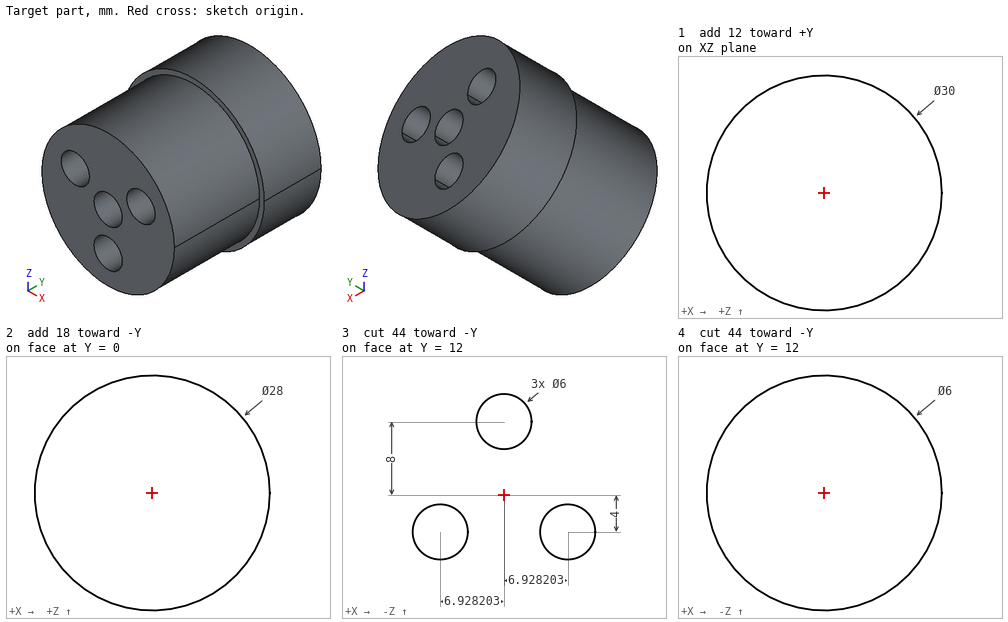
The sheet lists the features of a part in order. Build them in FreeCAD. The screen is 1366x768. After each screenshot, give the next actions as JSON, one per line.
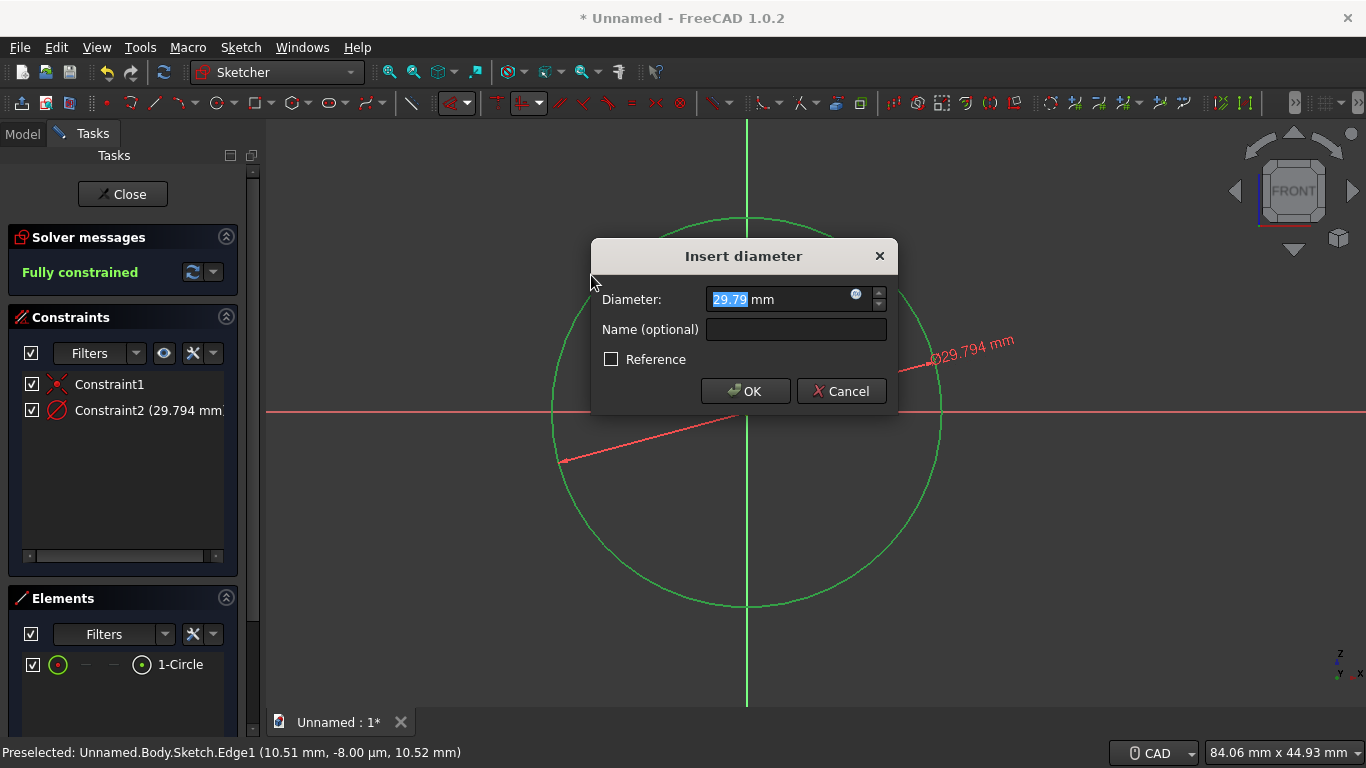
{"action": "type", "text": "30"}
{"action": "key", "text": "Return"}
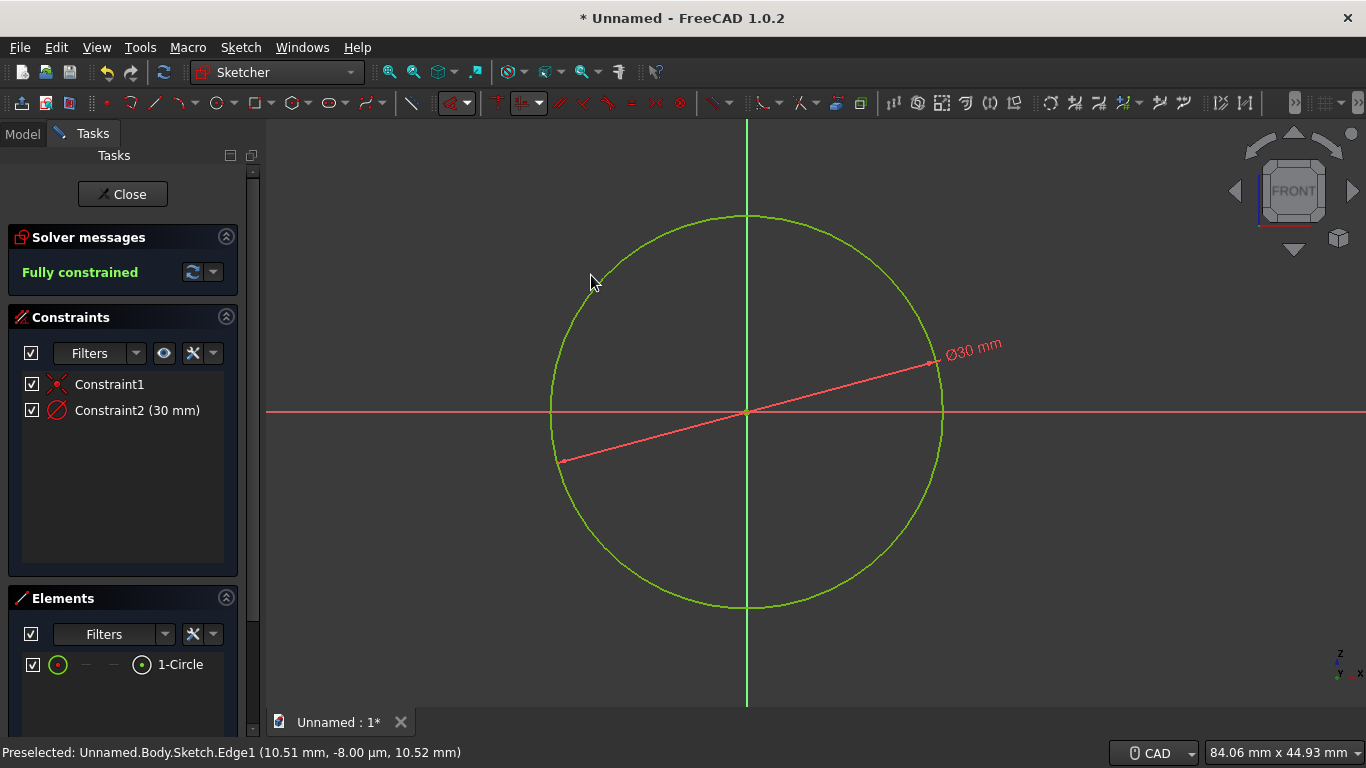
{"action": "left_click", "coordinate": [123, 194]}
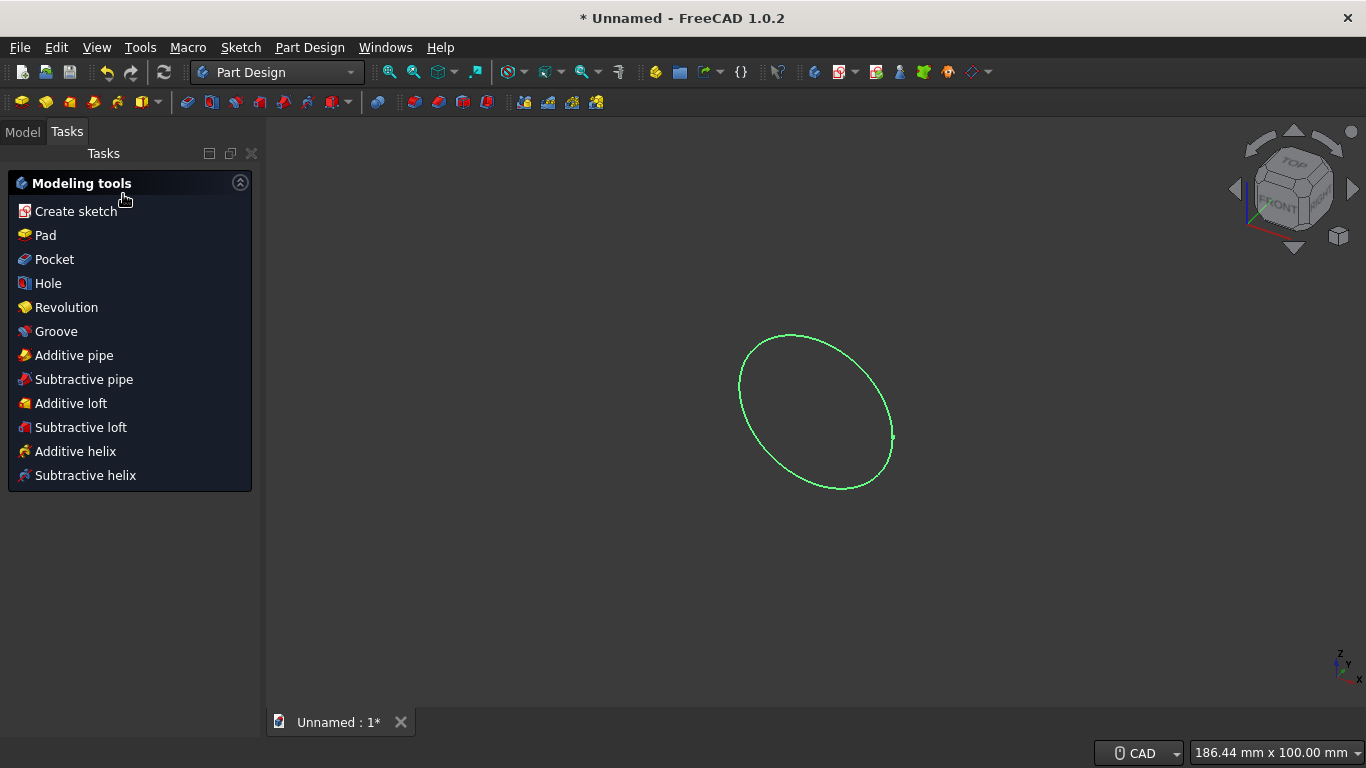
{"action": "left_click", "coordinate": [22, 102]}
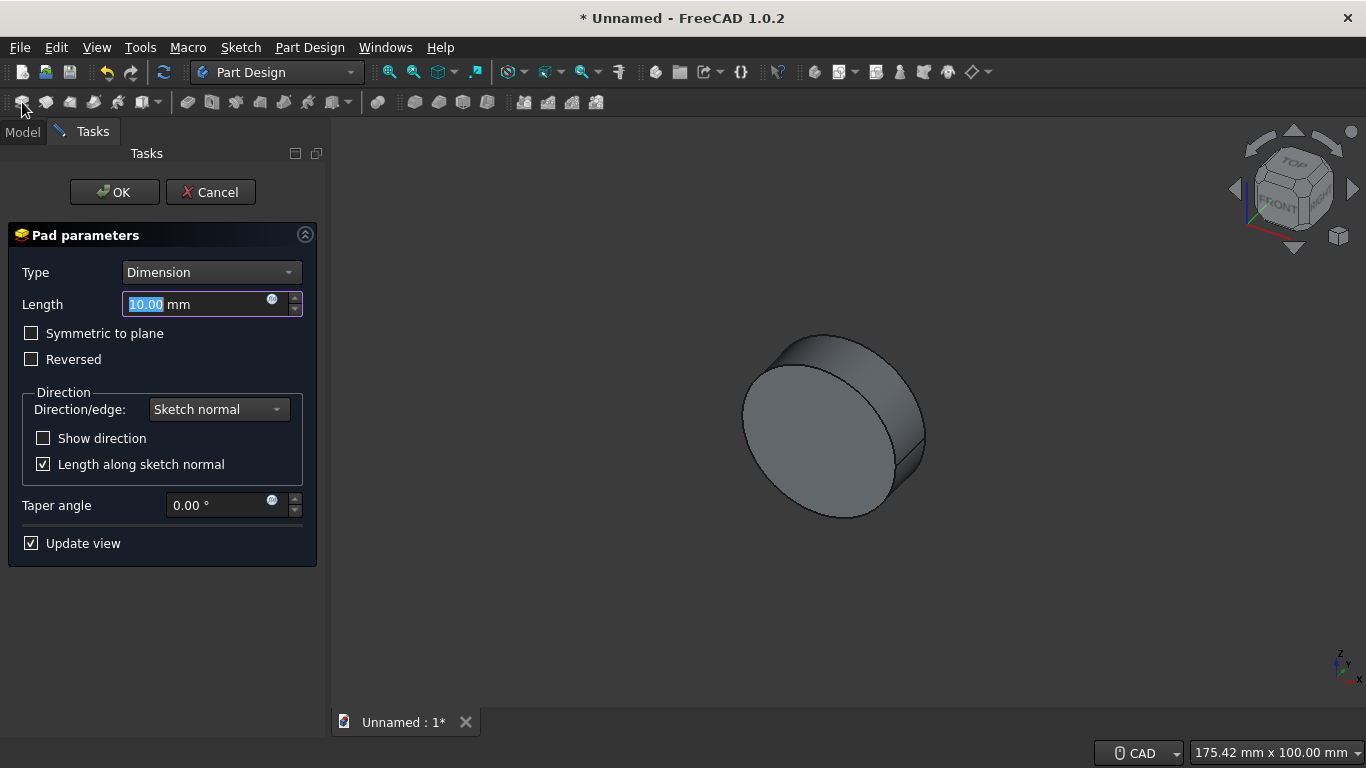
{"action": "type", "text": "12"}
{"action": "key", "text": "Tab"}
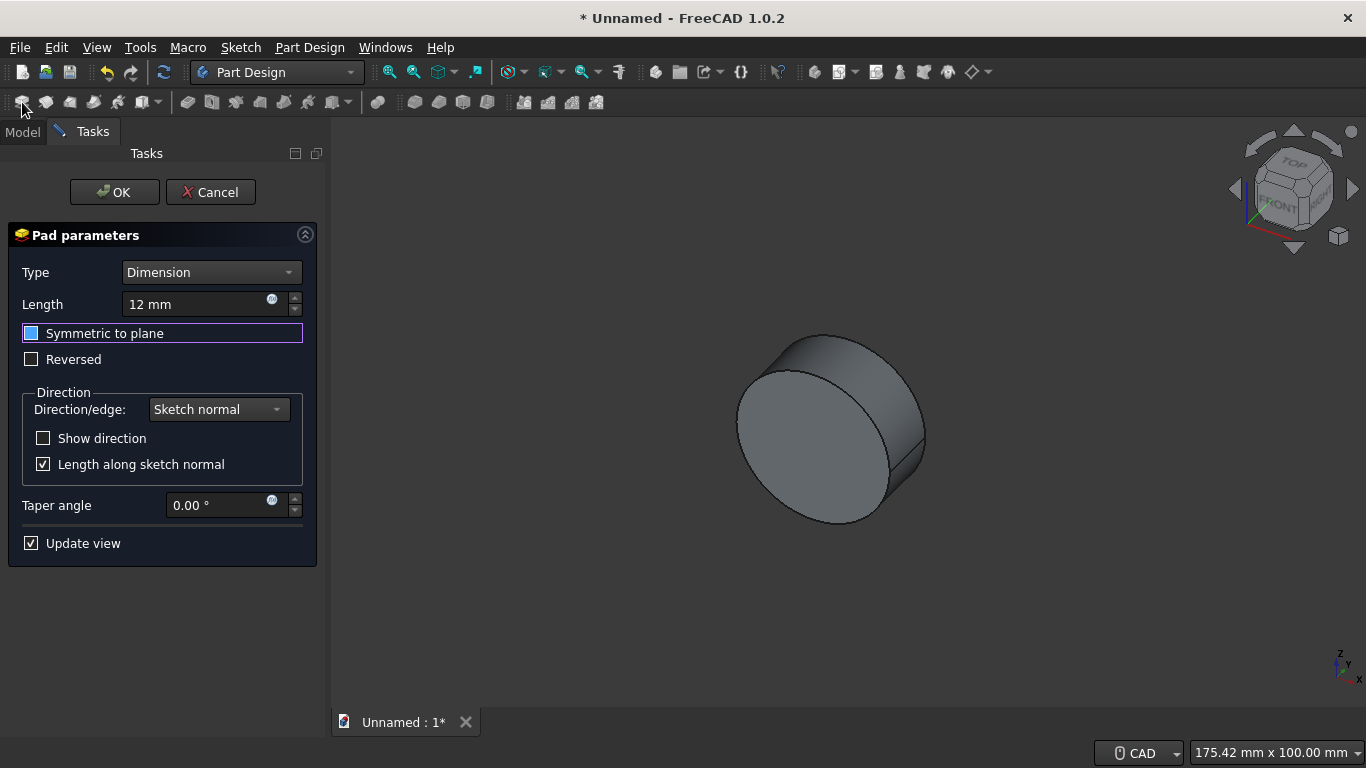
{"action": "left_click", "coordinate": [30, 359]}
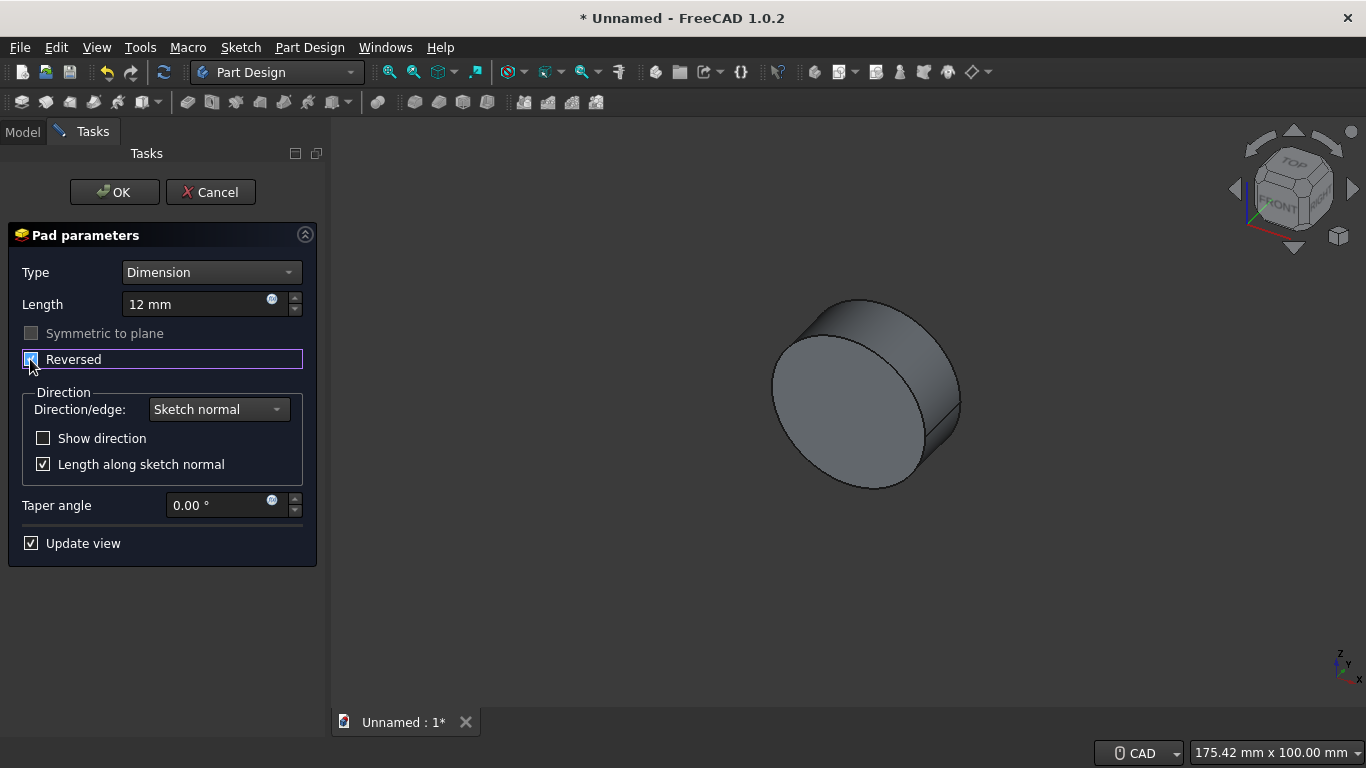
{"action": "left_click", "coordinate": [115, 192]}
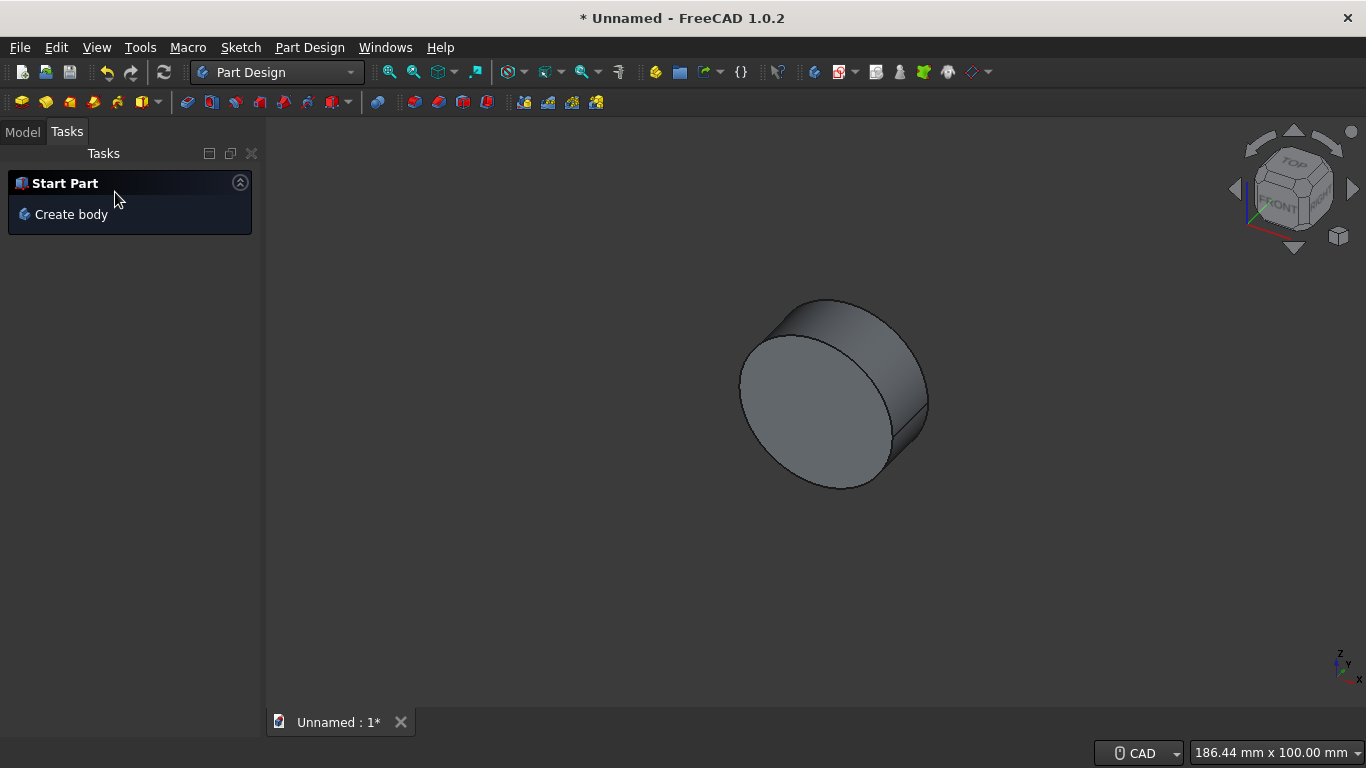
{"action": "left_click", "coordinate": [390, 72]}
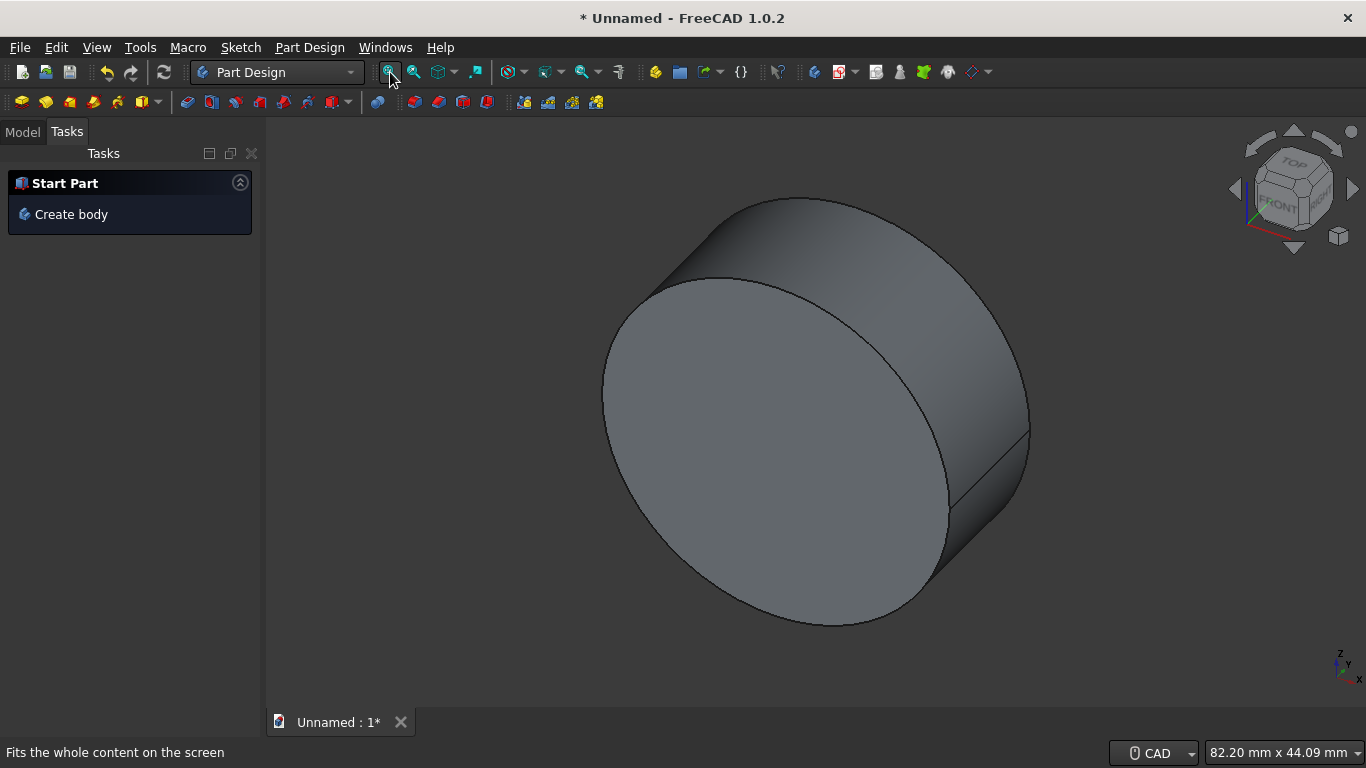
{"action": "left_click", "coordinate": [776, 451]}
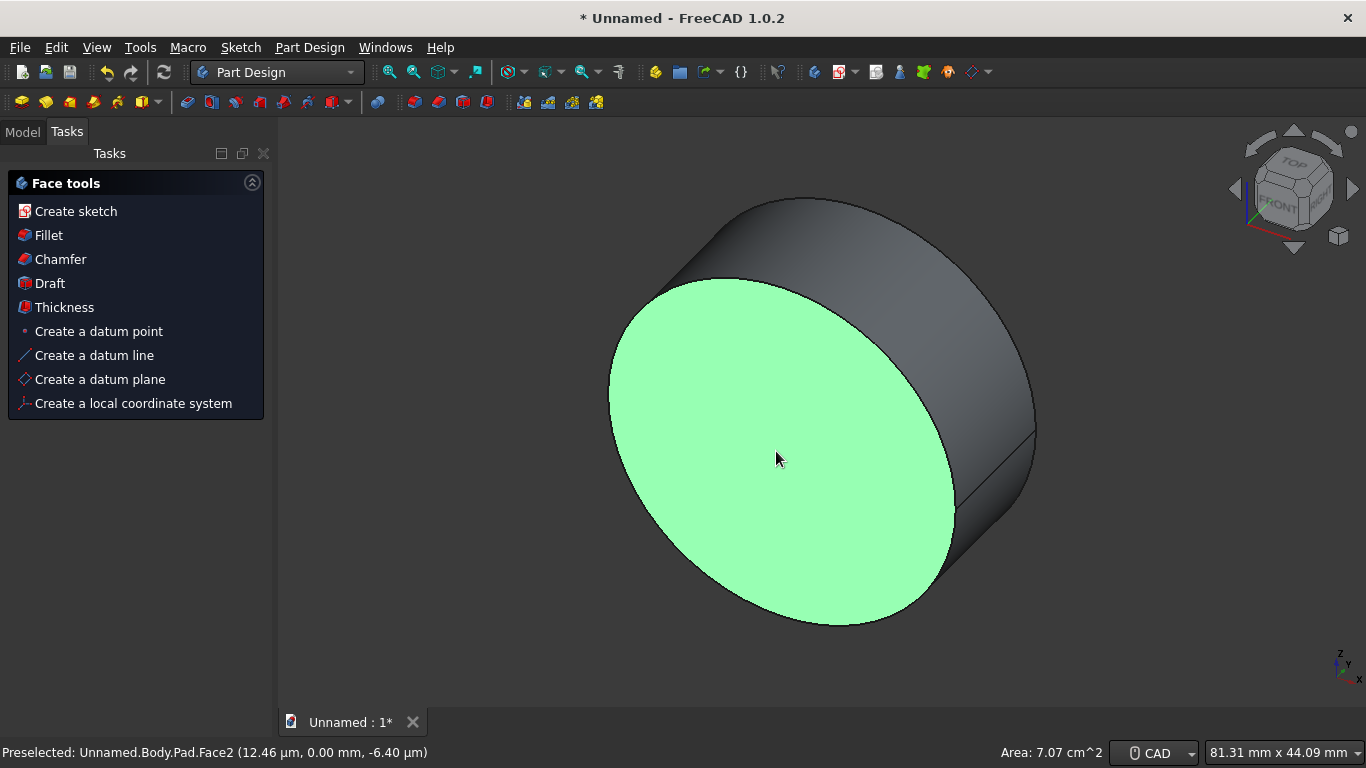
{"action": "left_click", "coordinate": [840, 72]}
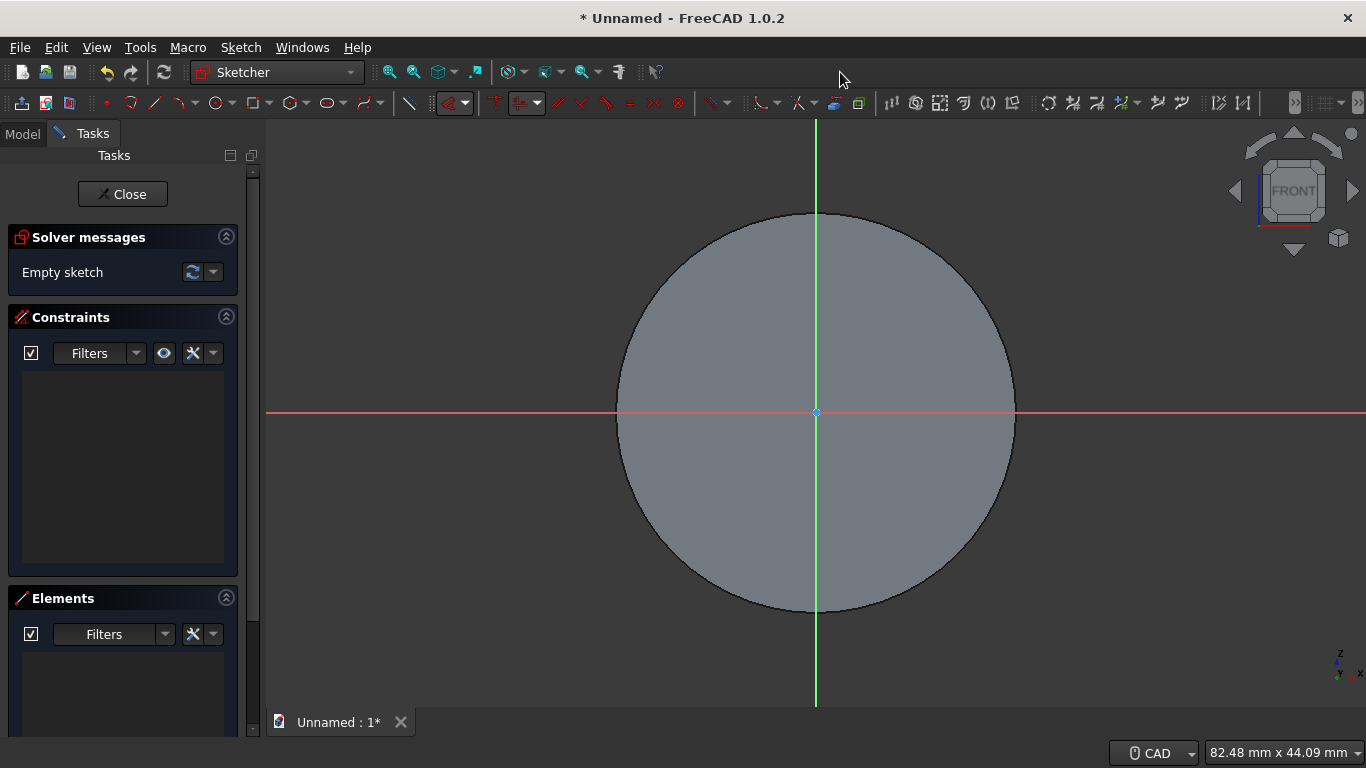
{"action": "left_click", "coordinate": [216, 104]}